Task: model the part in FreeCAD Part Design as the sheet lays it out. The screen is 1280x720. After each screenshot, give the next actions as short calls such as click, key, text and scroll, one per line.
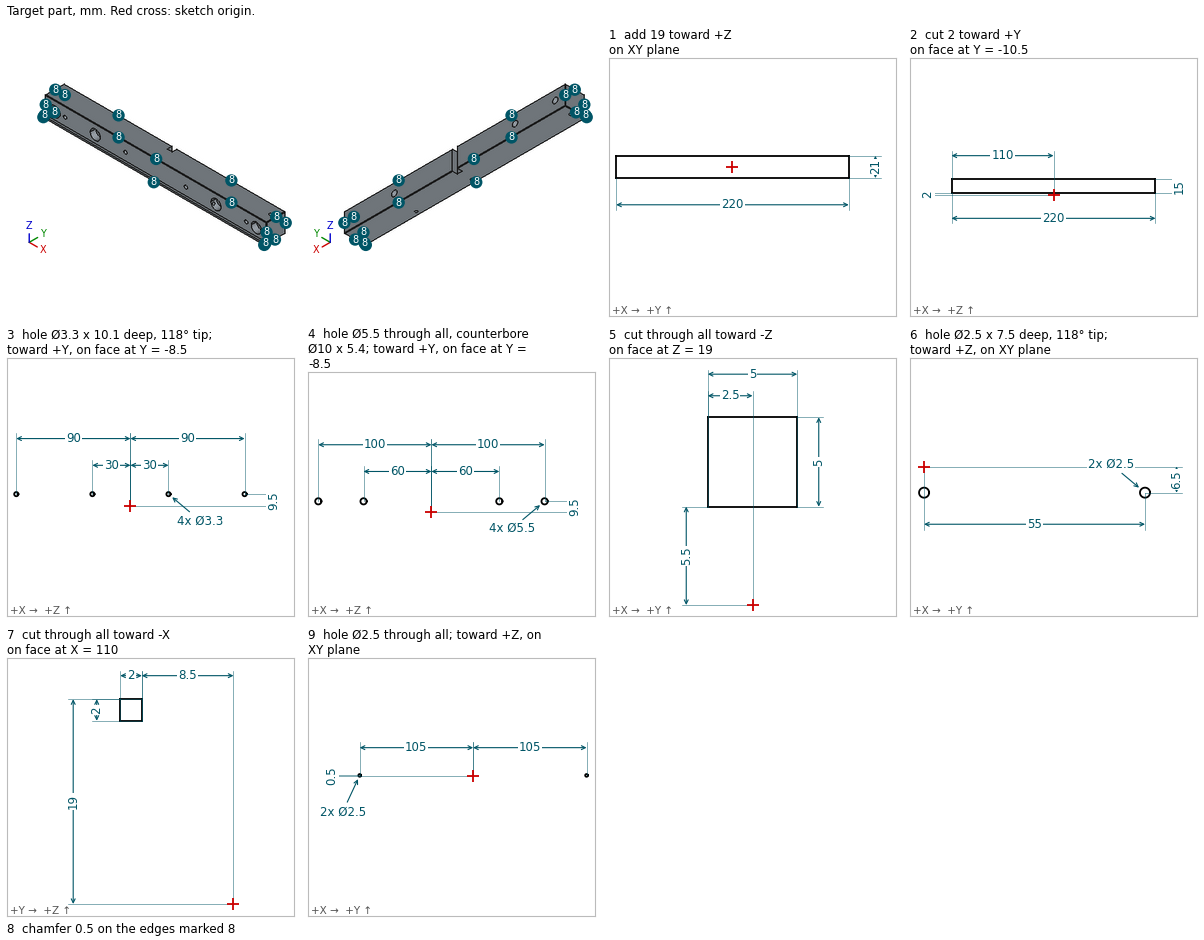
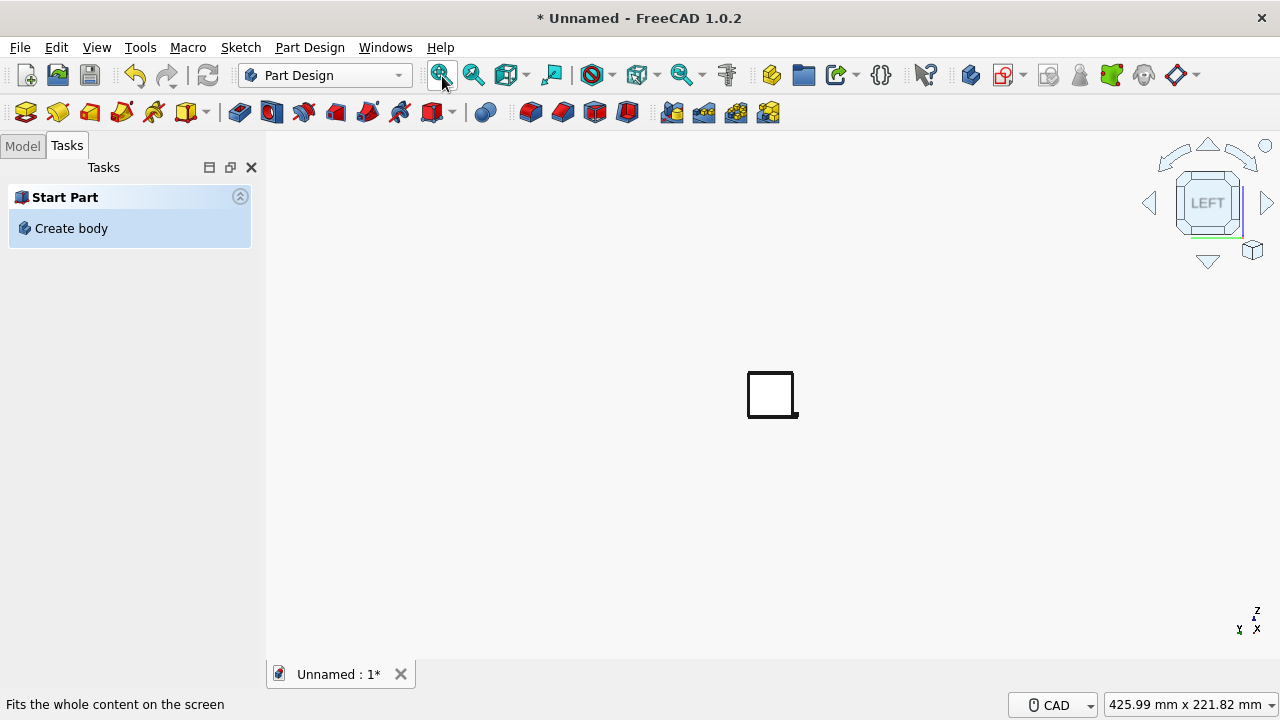
click(1004, 76)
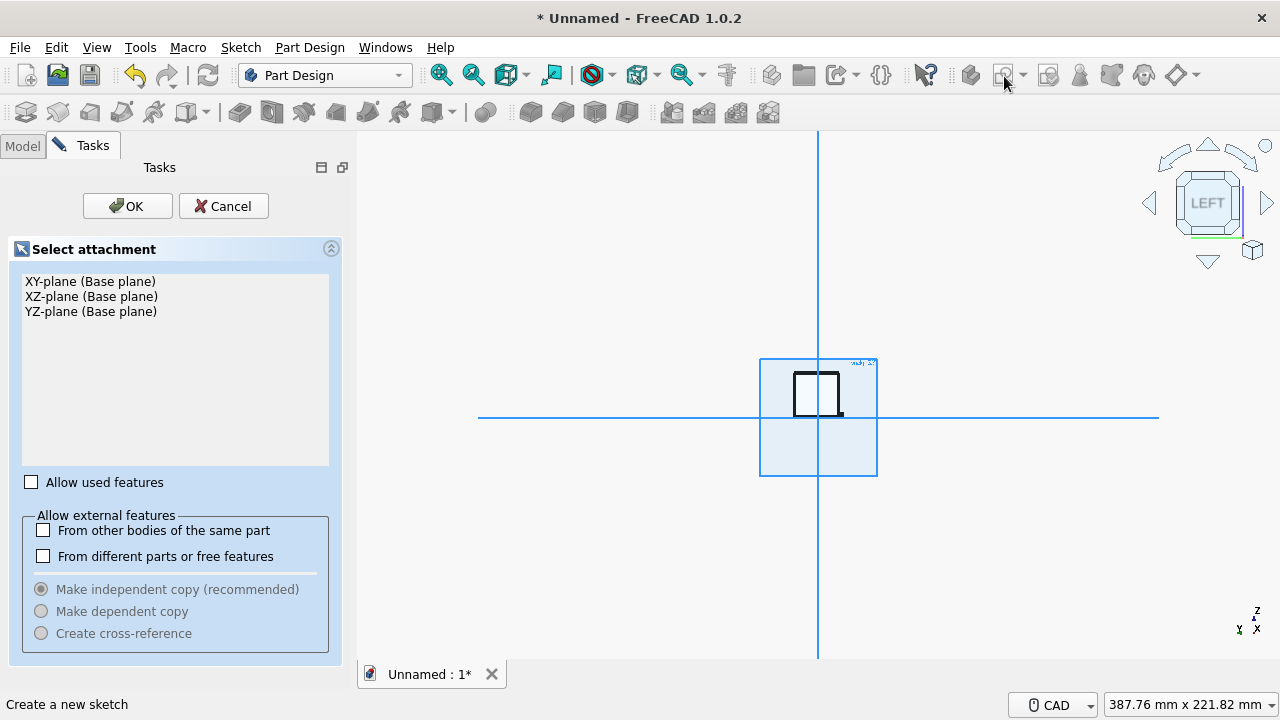
click(82, 282)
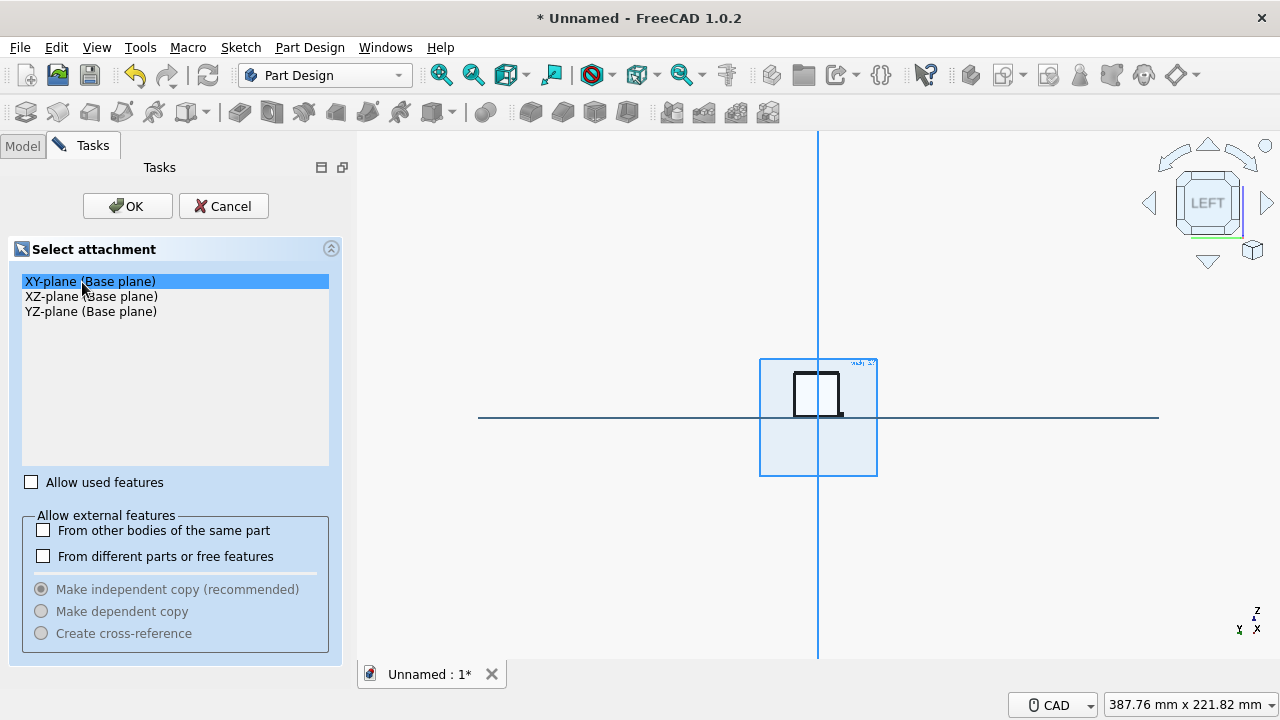
click(128, 206)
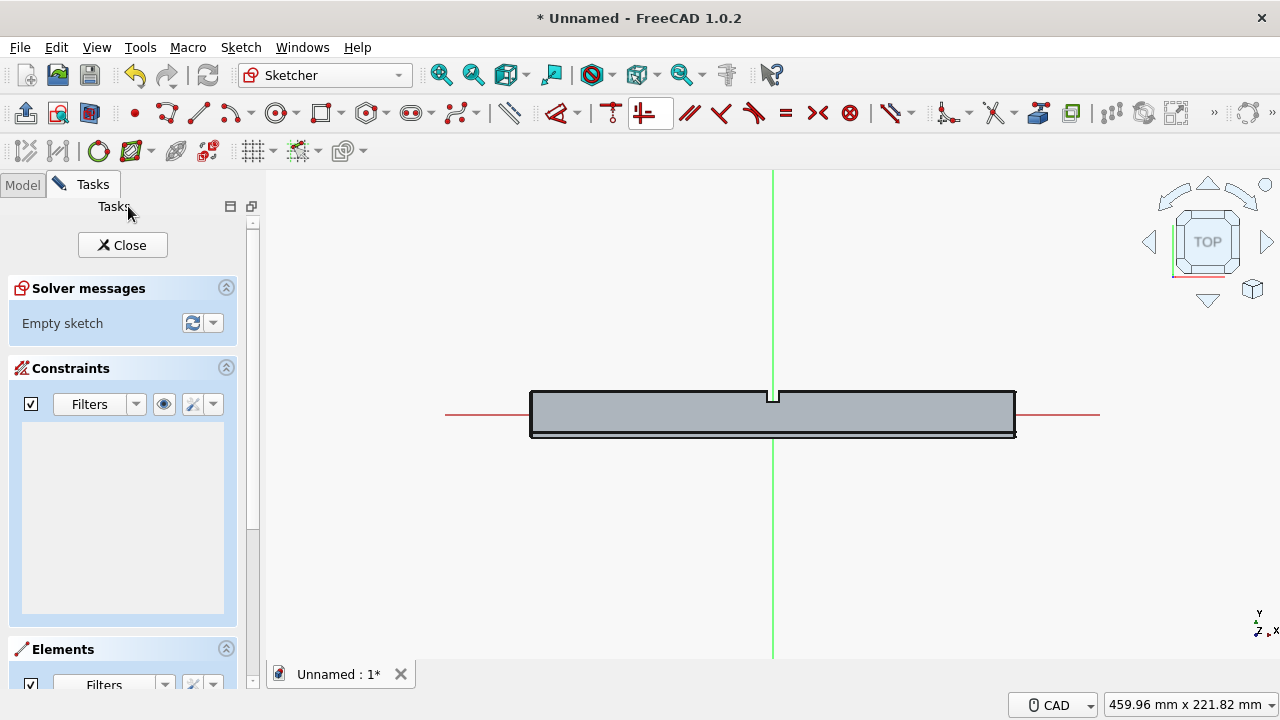
click(90, 114)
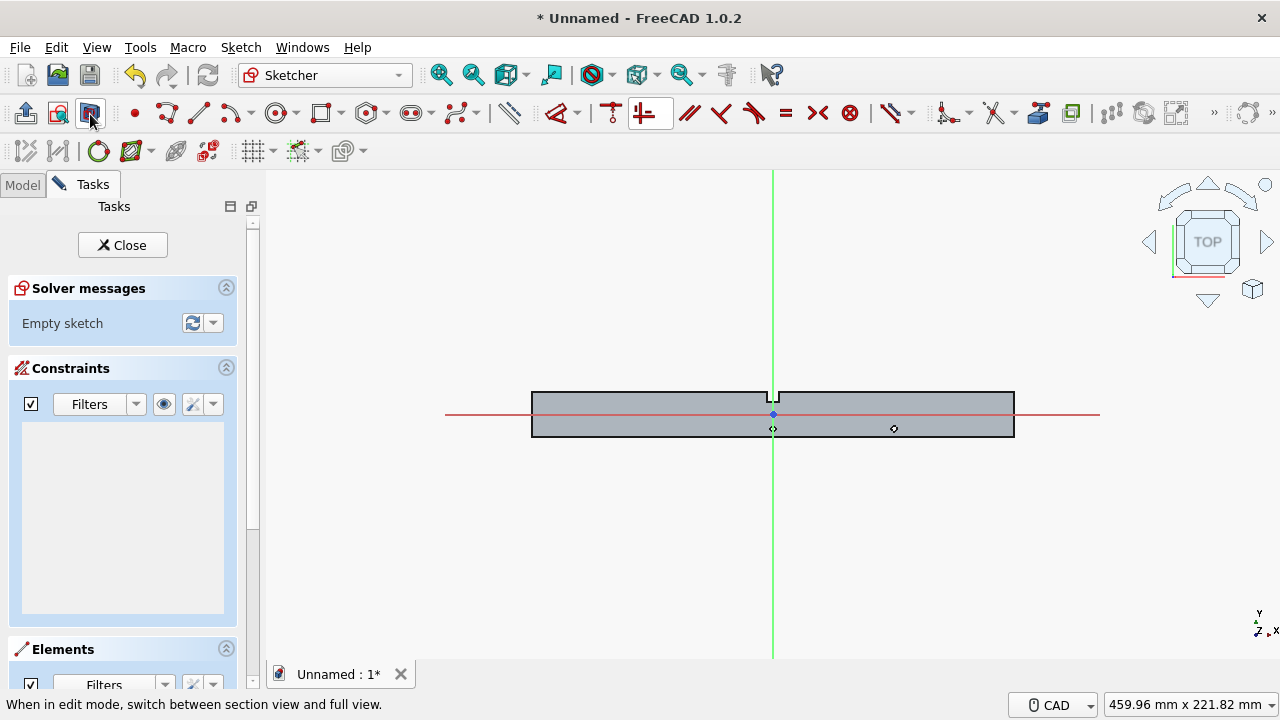
click(276, 114)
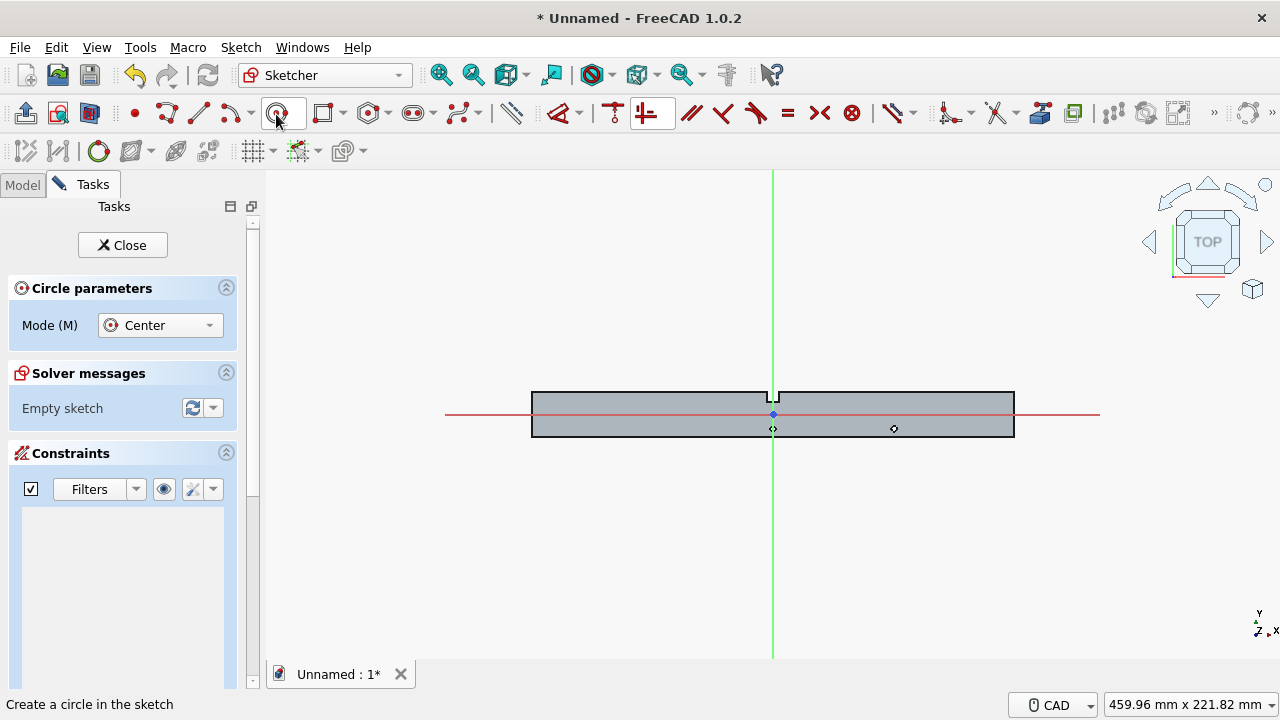
scroll(542, 413, up, 14)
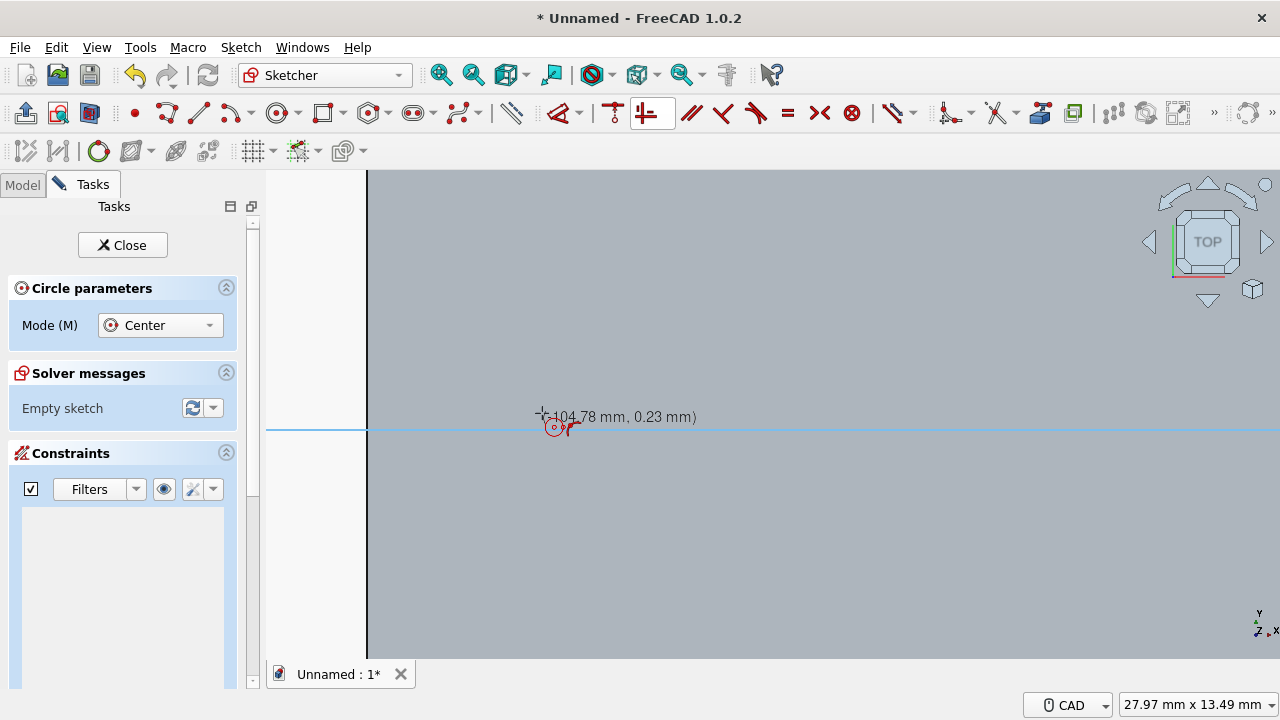
click(530, 412)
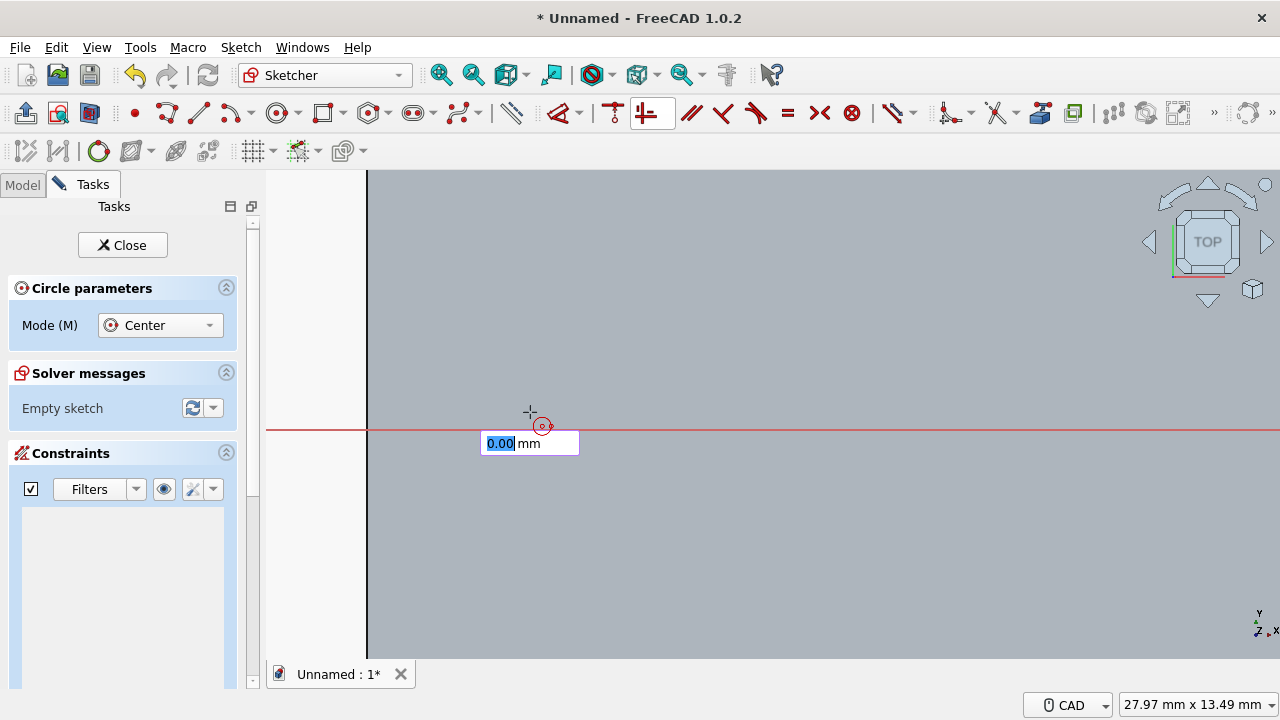
scroll(413, 415, down, 13)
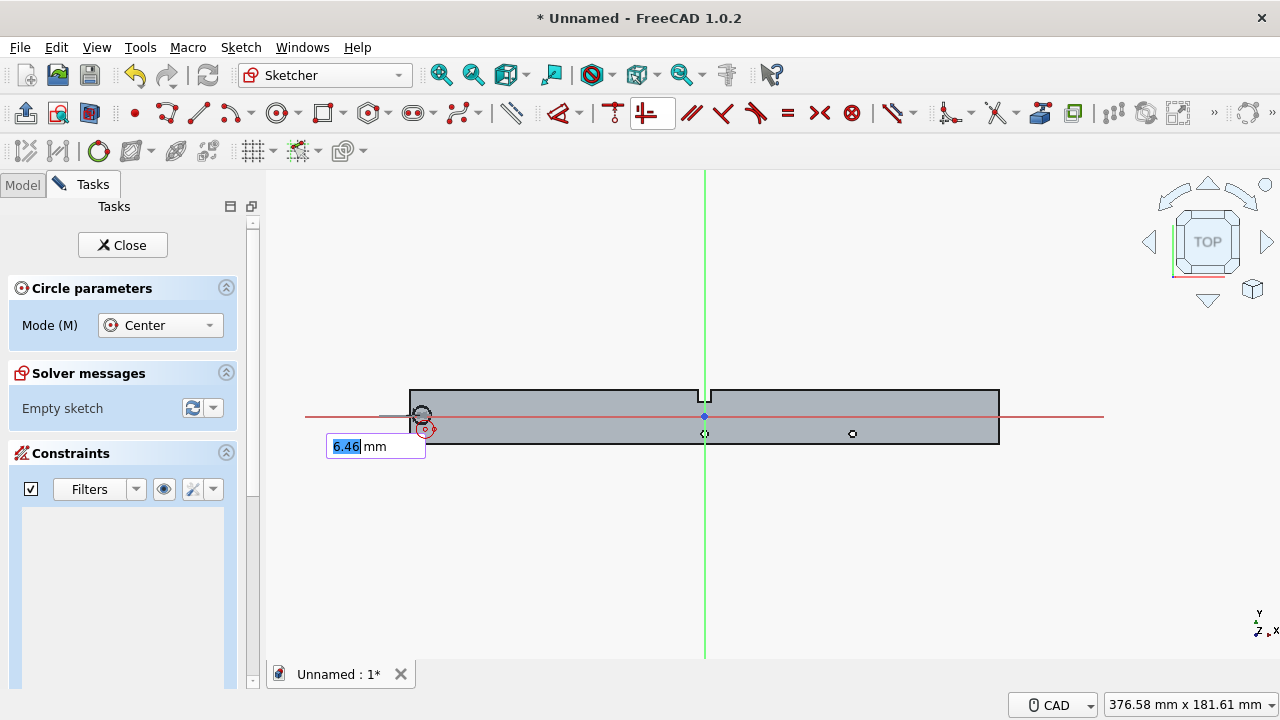
scroll(424, 413, up, 8)
move(424, 410)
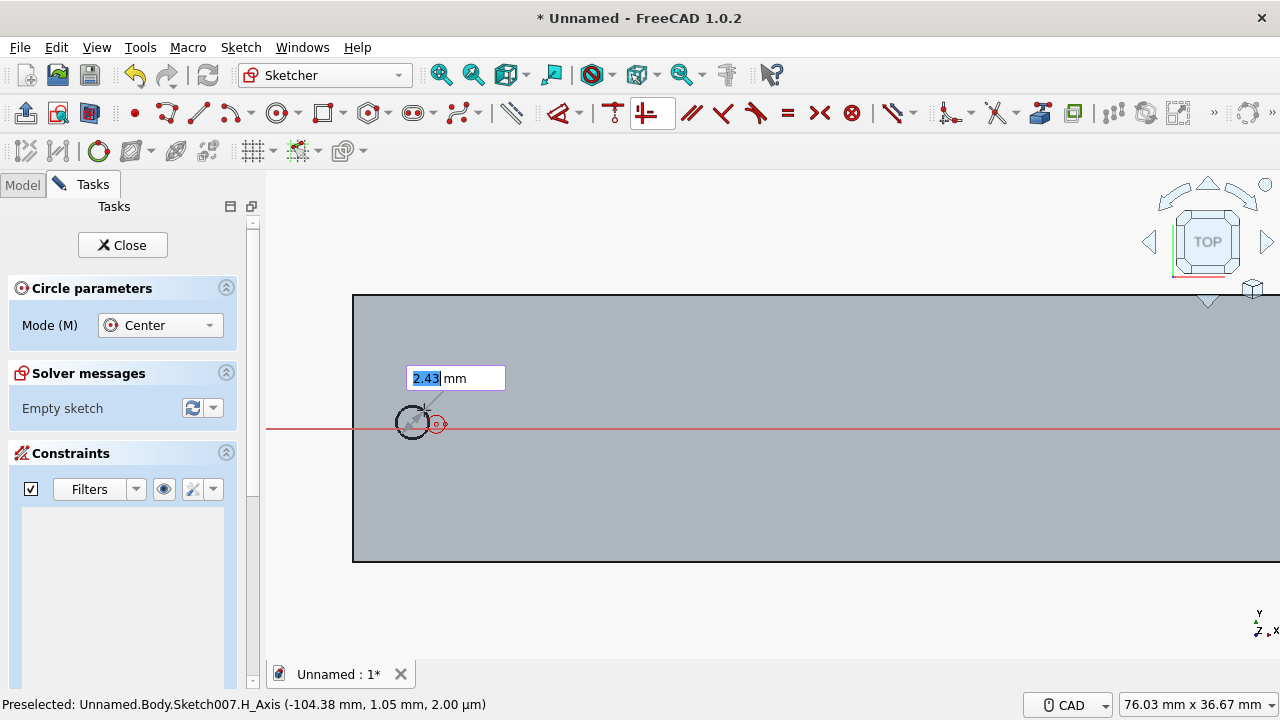
text(2.5)
key(Return)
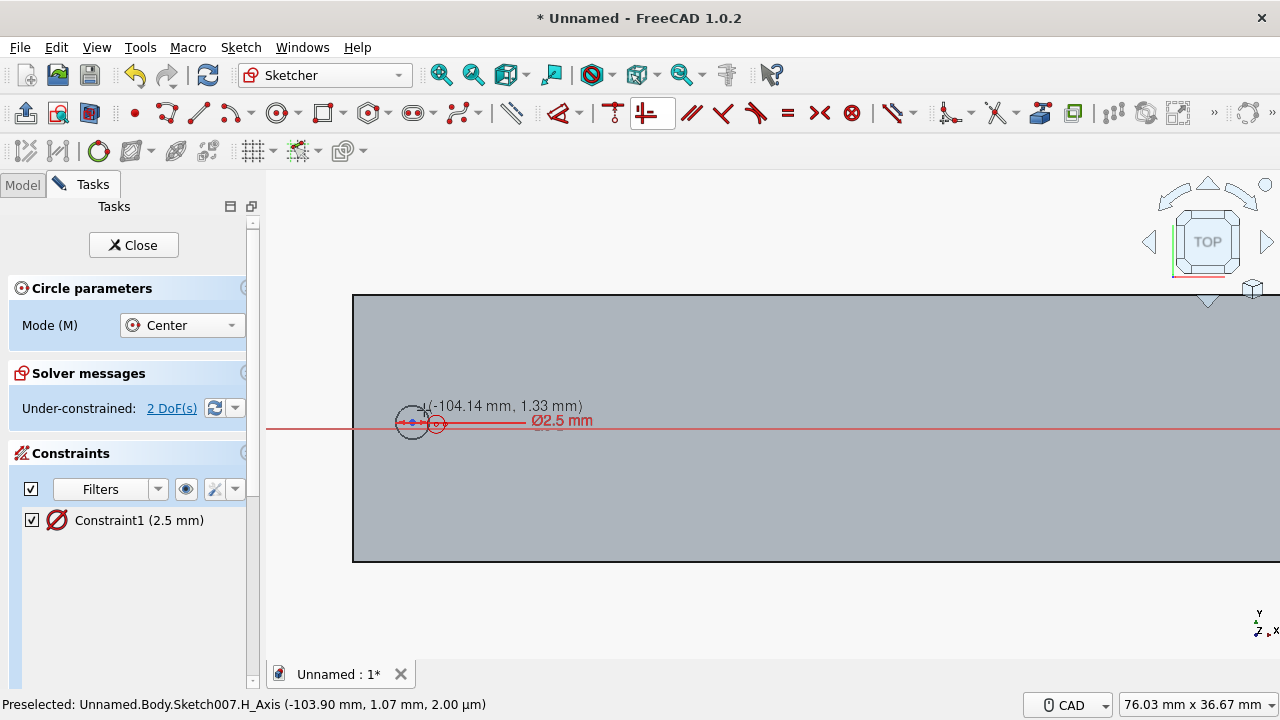
scroll(424, 413, down, 8)